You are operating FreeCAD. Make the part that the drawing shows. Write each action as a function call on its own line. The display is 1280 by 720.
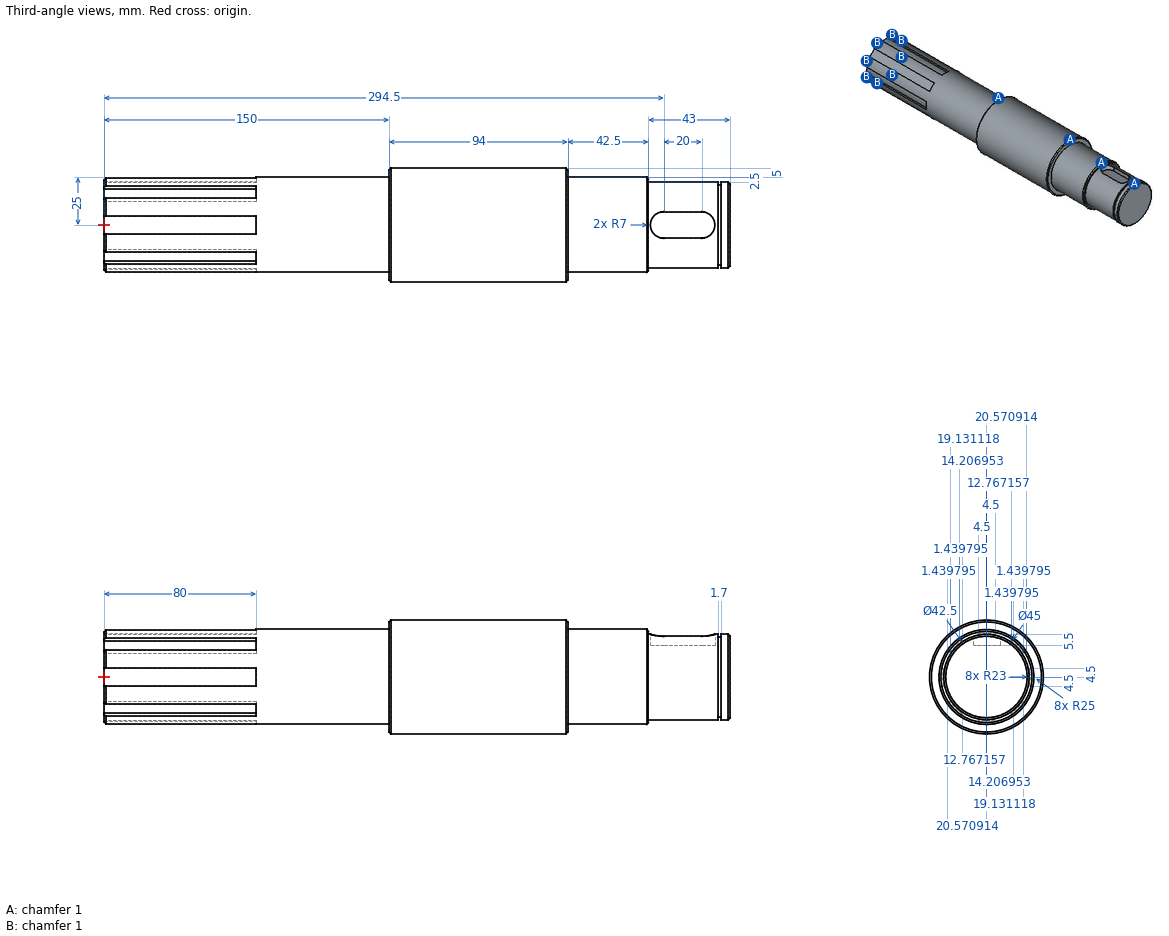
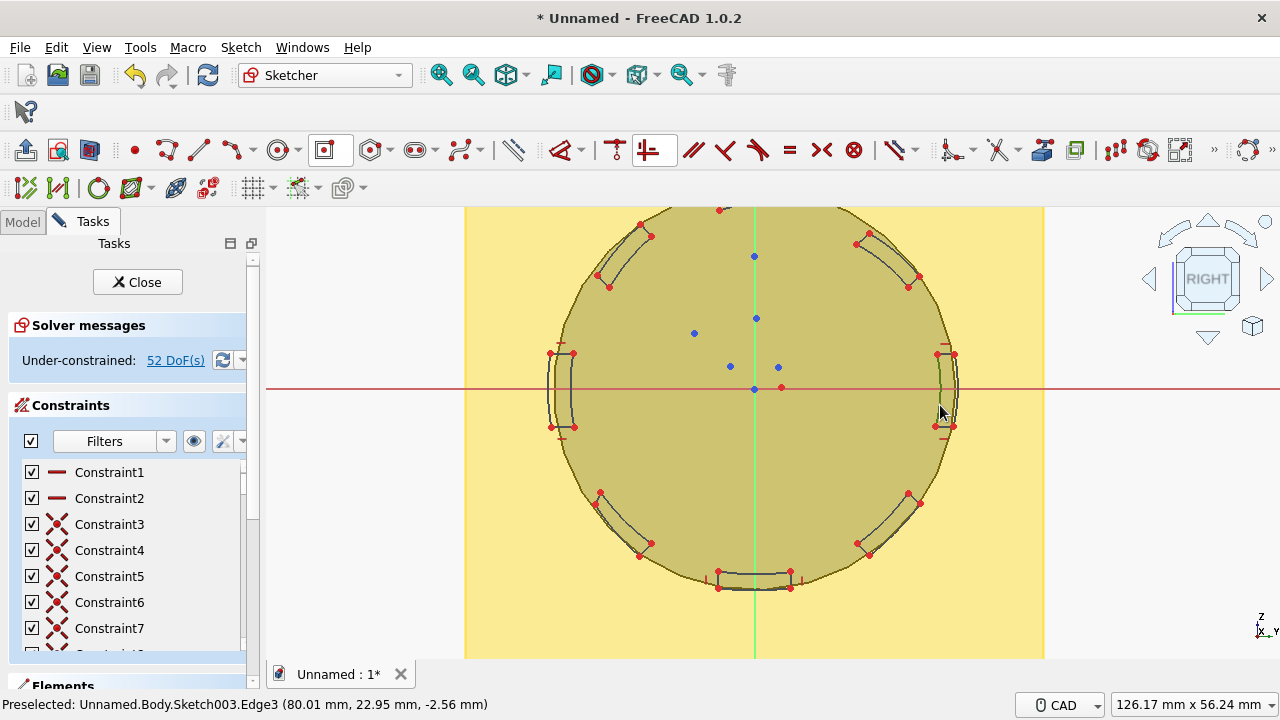
click(614, 510)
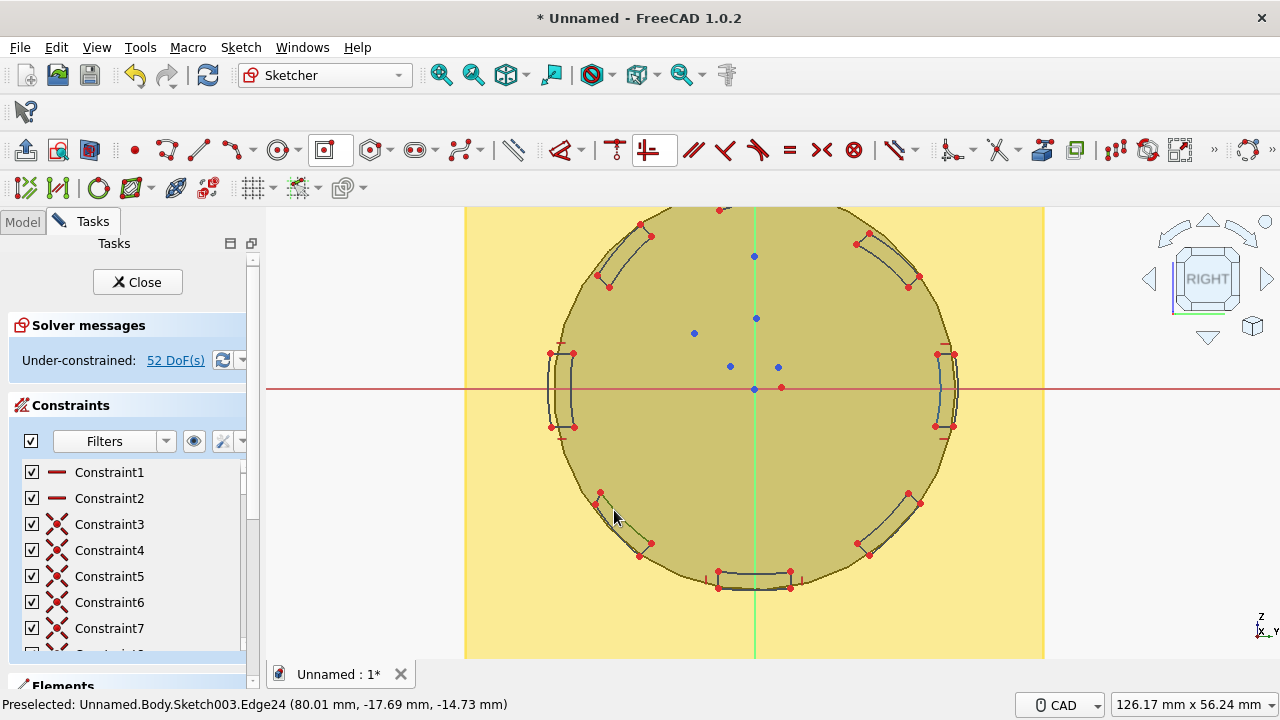
click(616, 150)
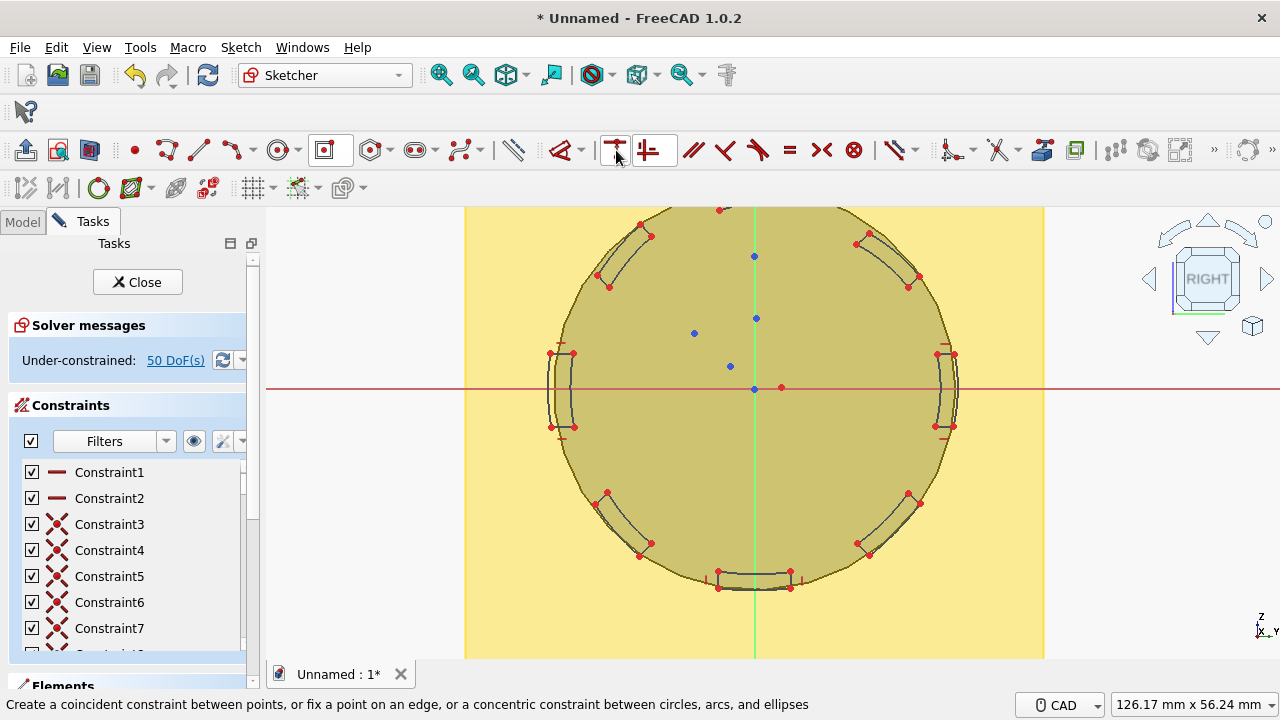
click(940, 405)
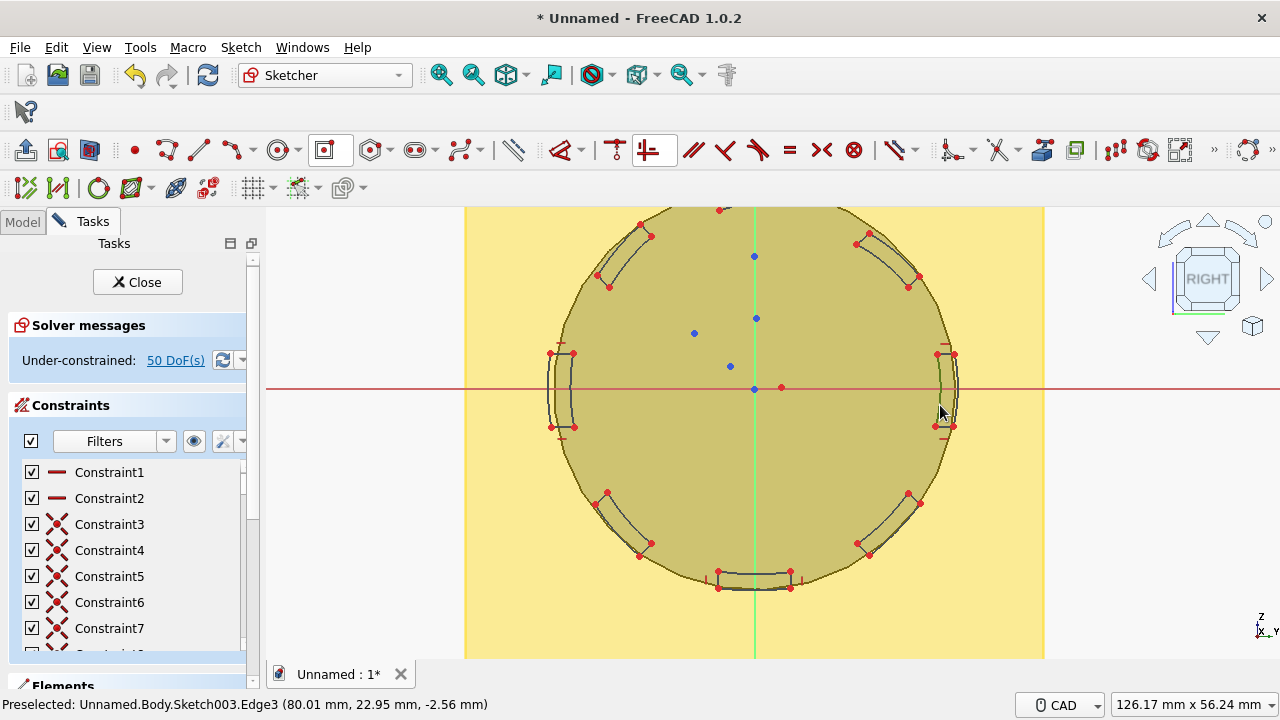
click(740, 590)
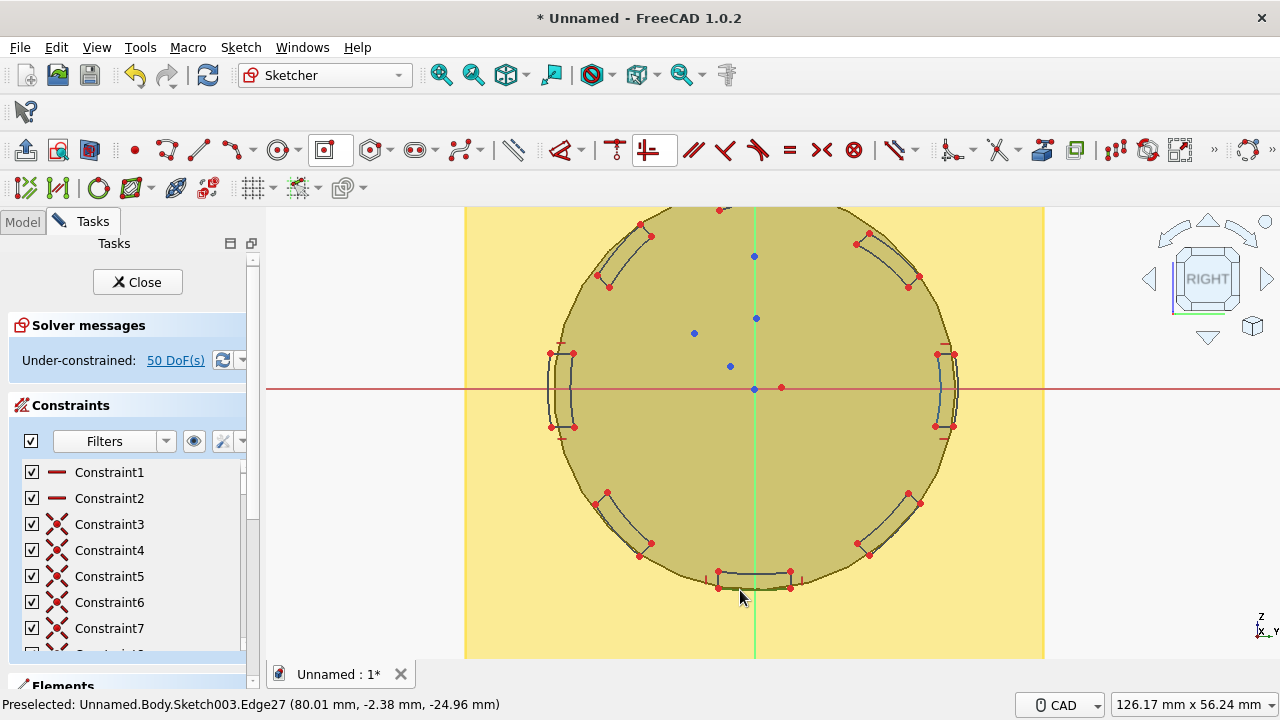
click(616, 150)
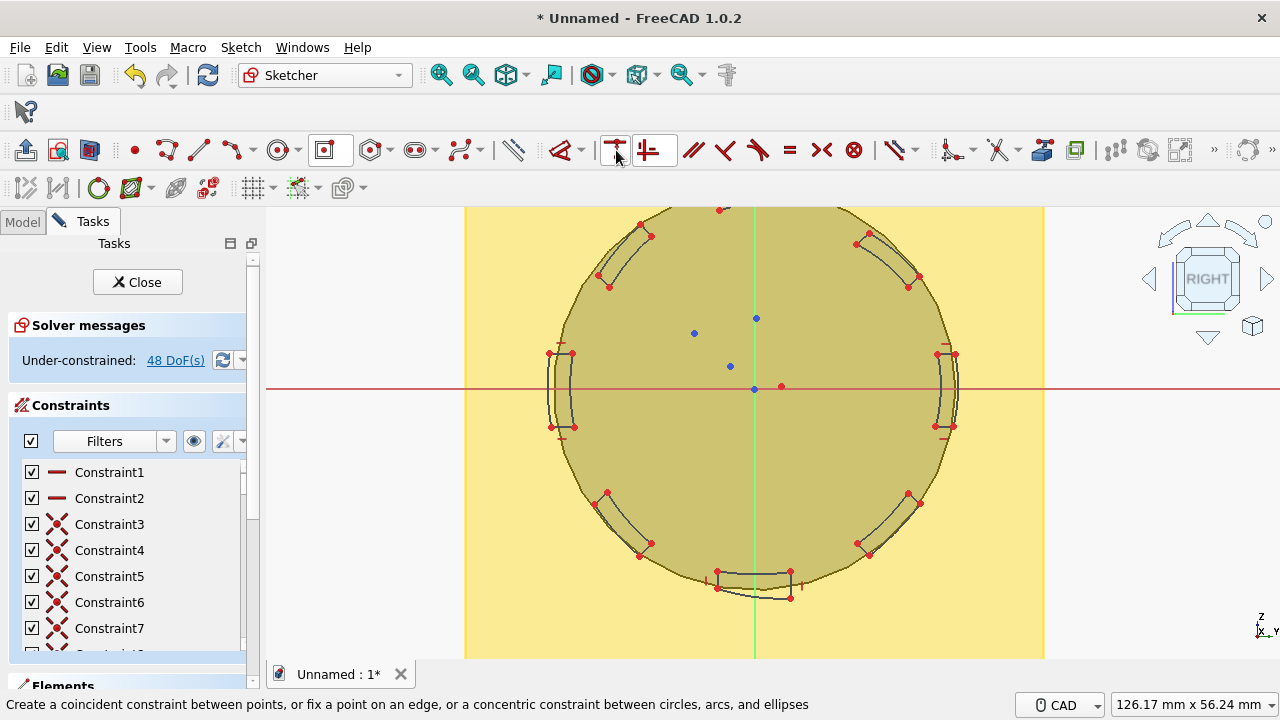
click(940, 405)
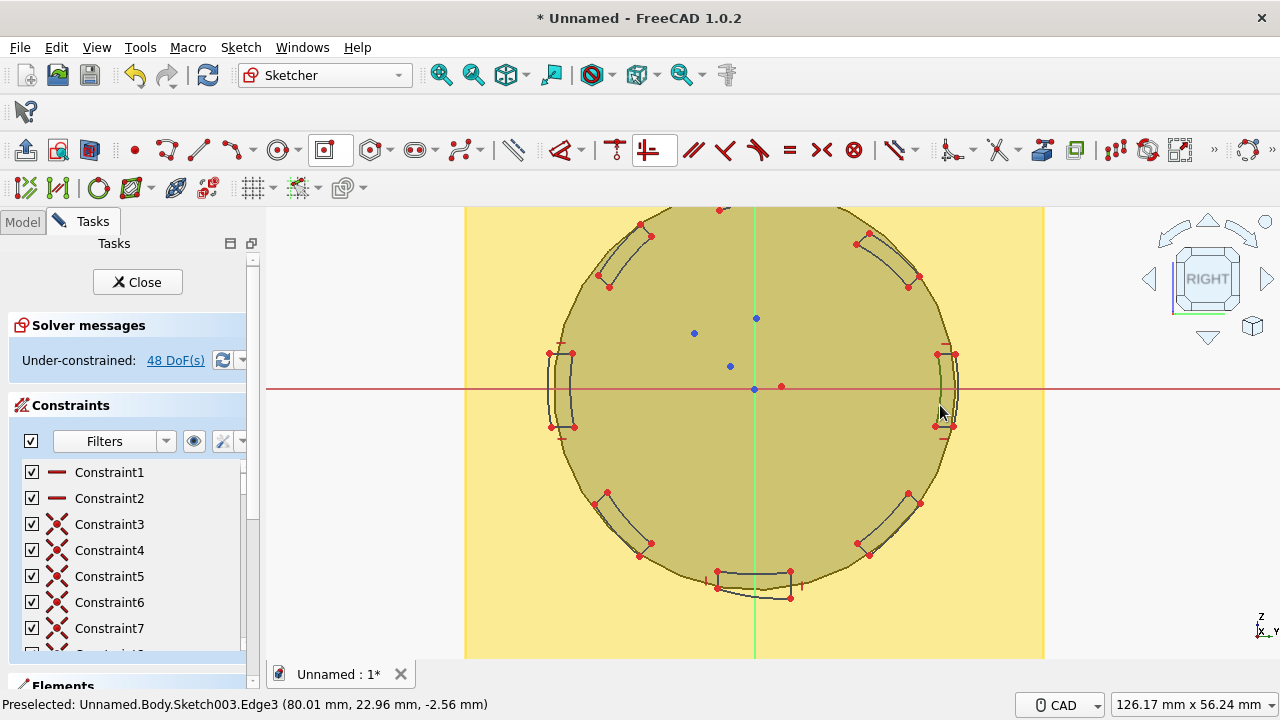
click(740, 574)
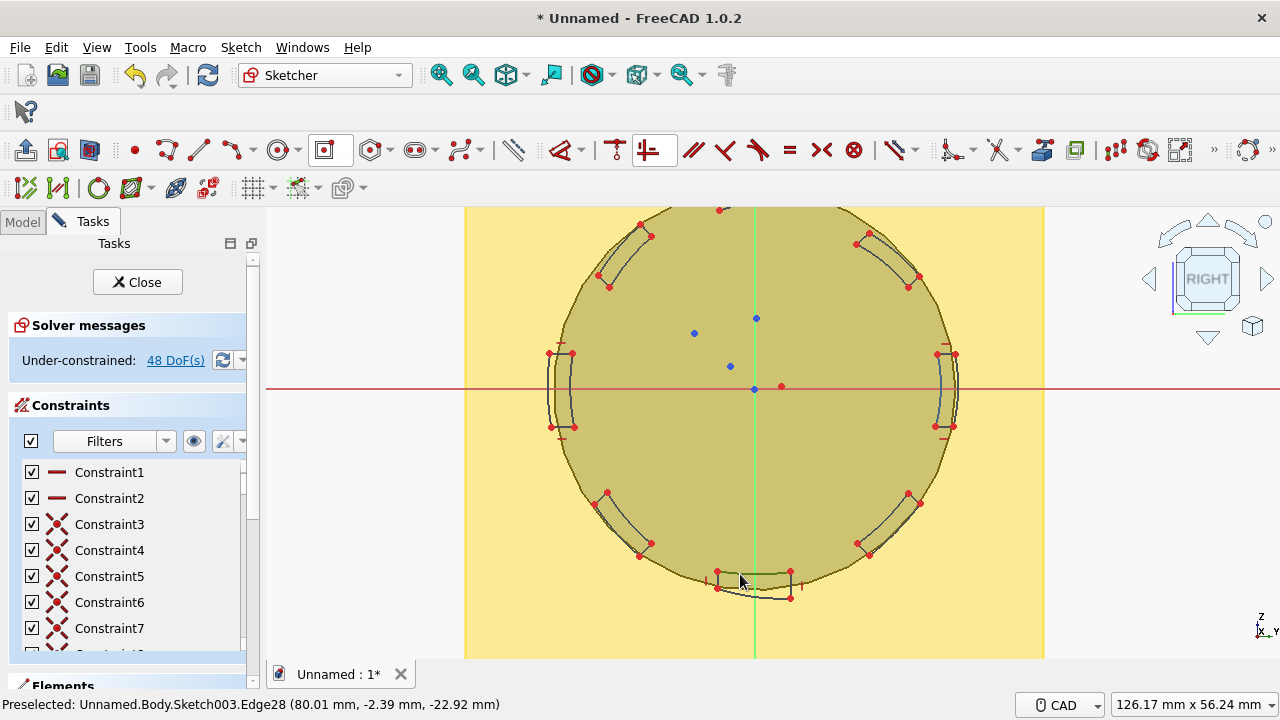
click(616, 150)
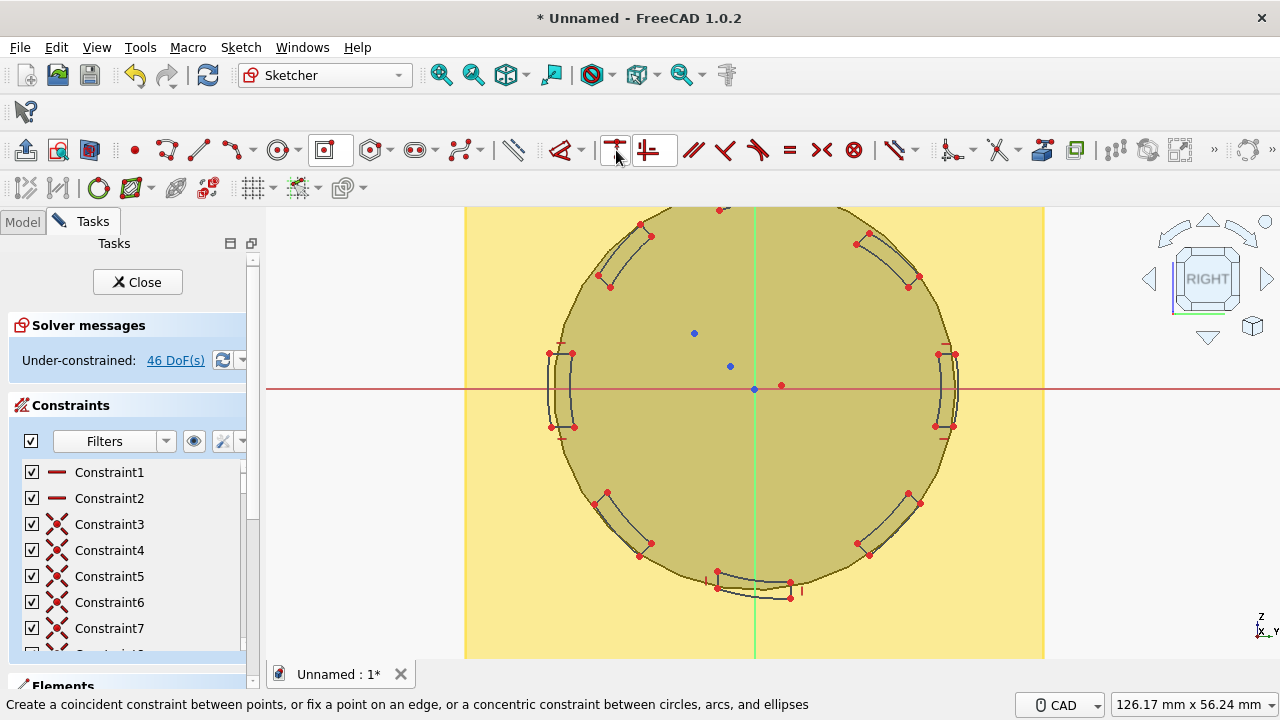
click(940, 405)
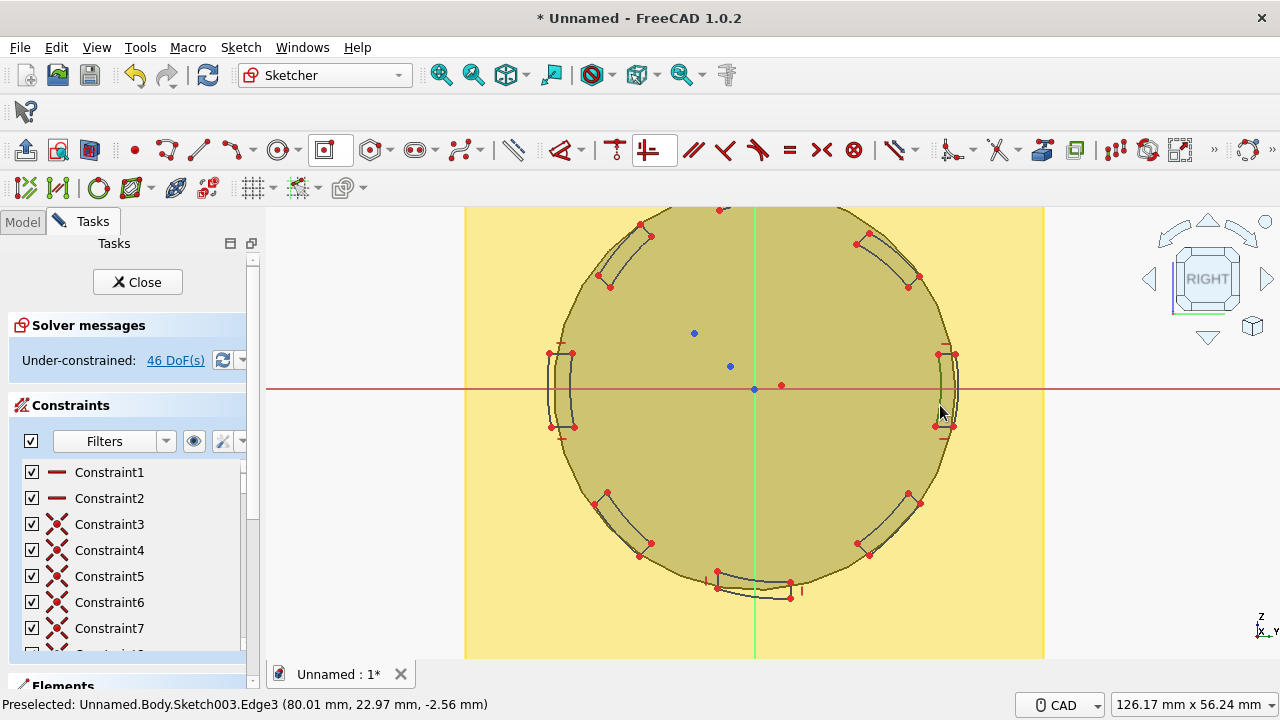
click(886, 542)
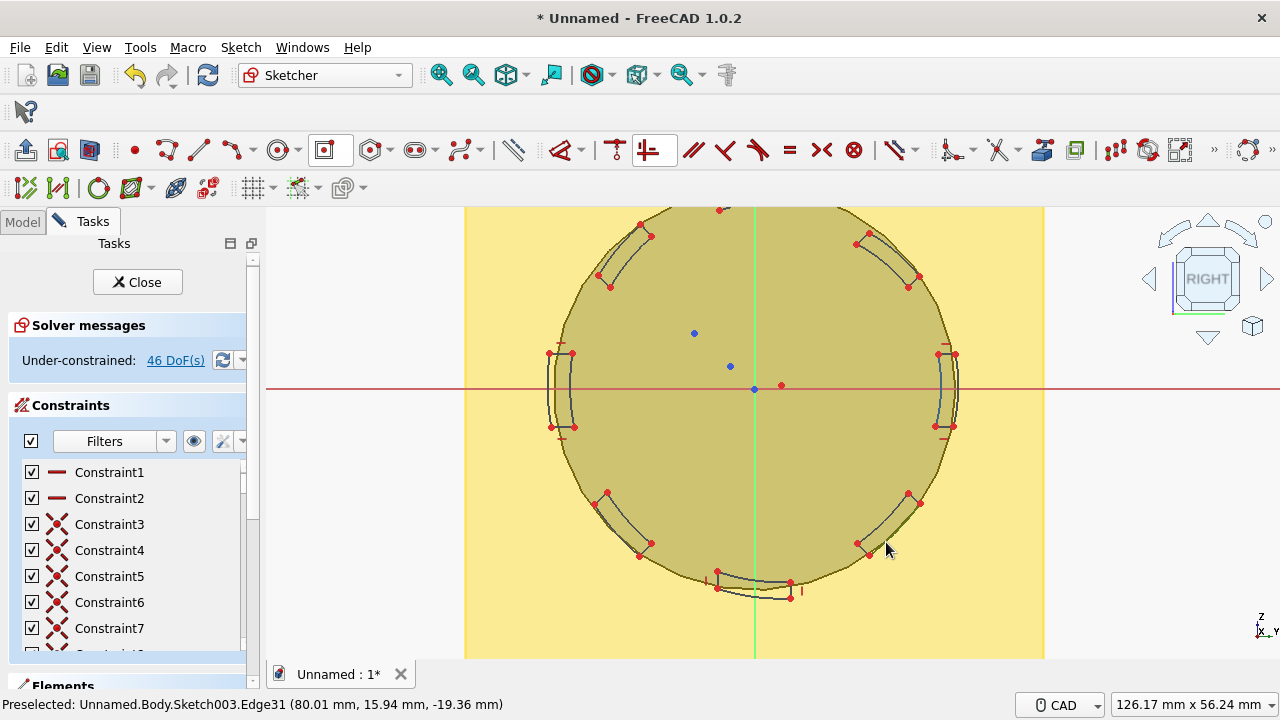
click(616, 150)